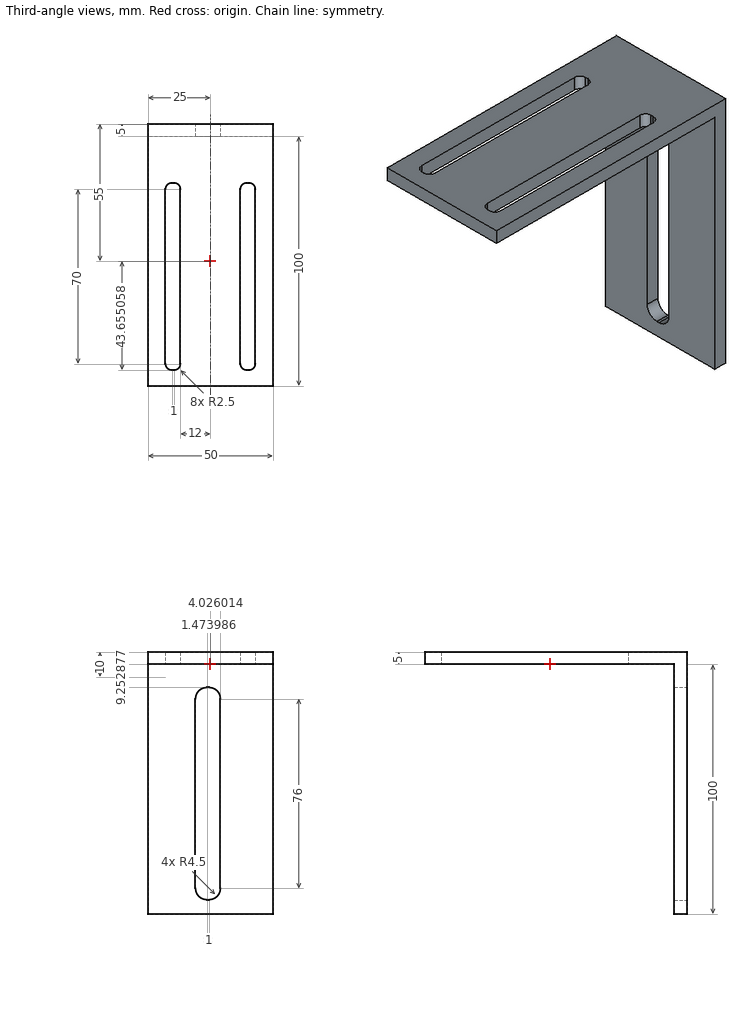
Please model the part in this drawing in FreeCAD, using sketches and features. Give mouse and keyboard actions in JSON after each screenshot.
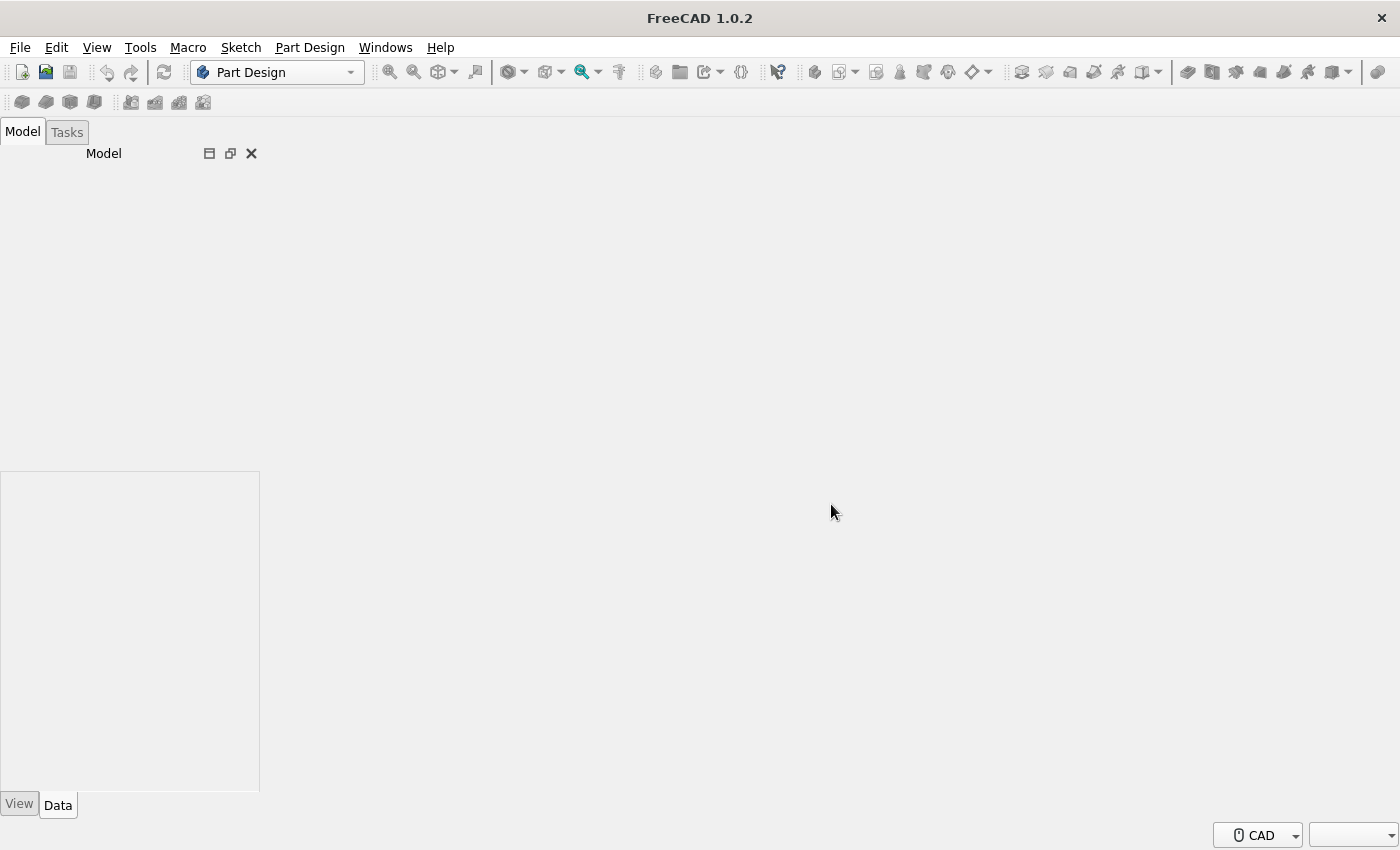
{"action": "left_click", "coordinate": [22, 72]}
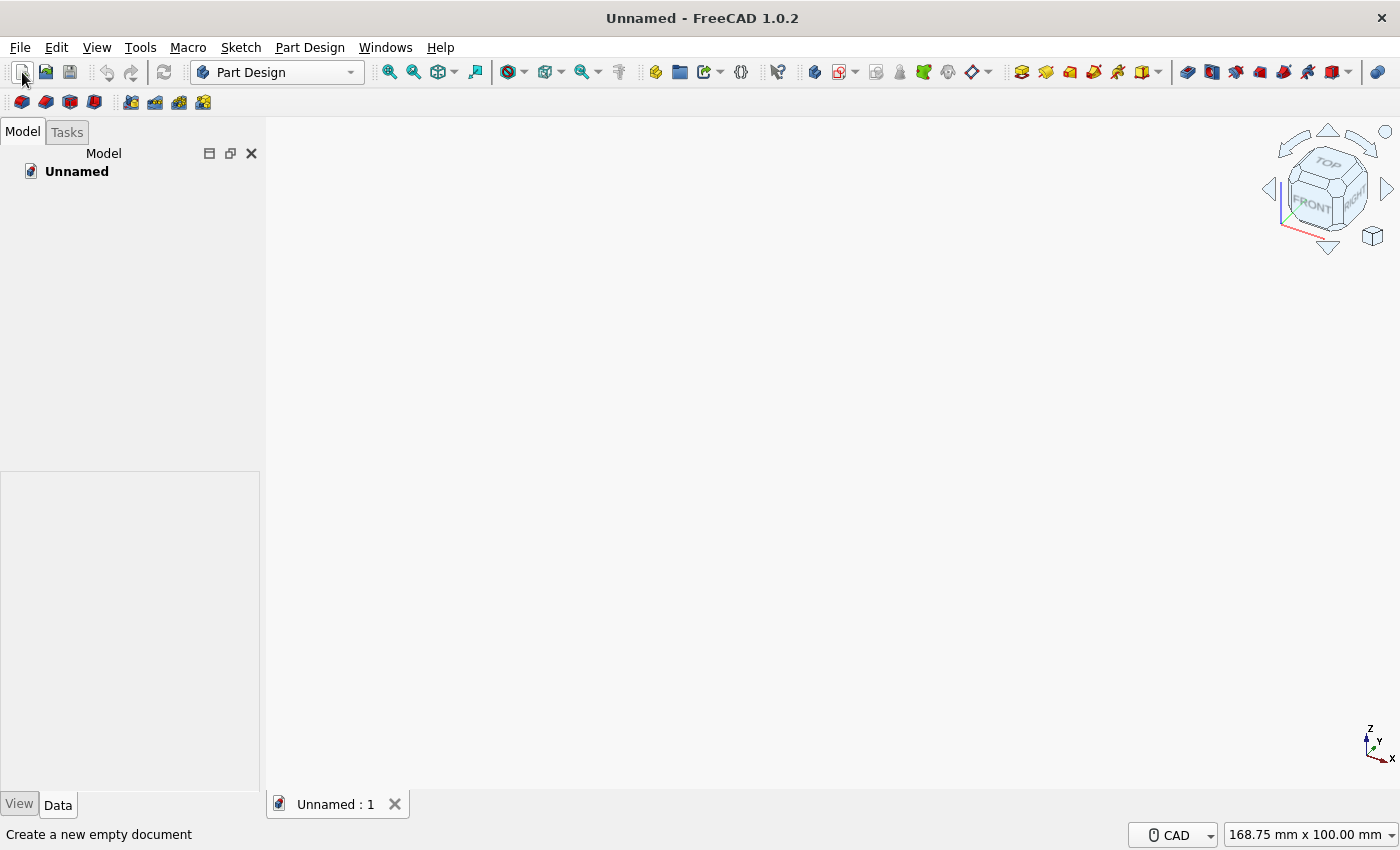
{"action": "left_click", "coordinate": [840, 72]}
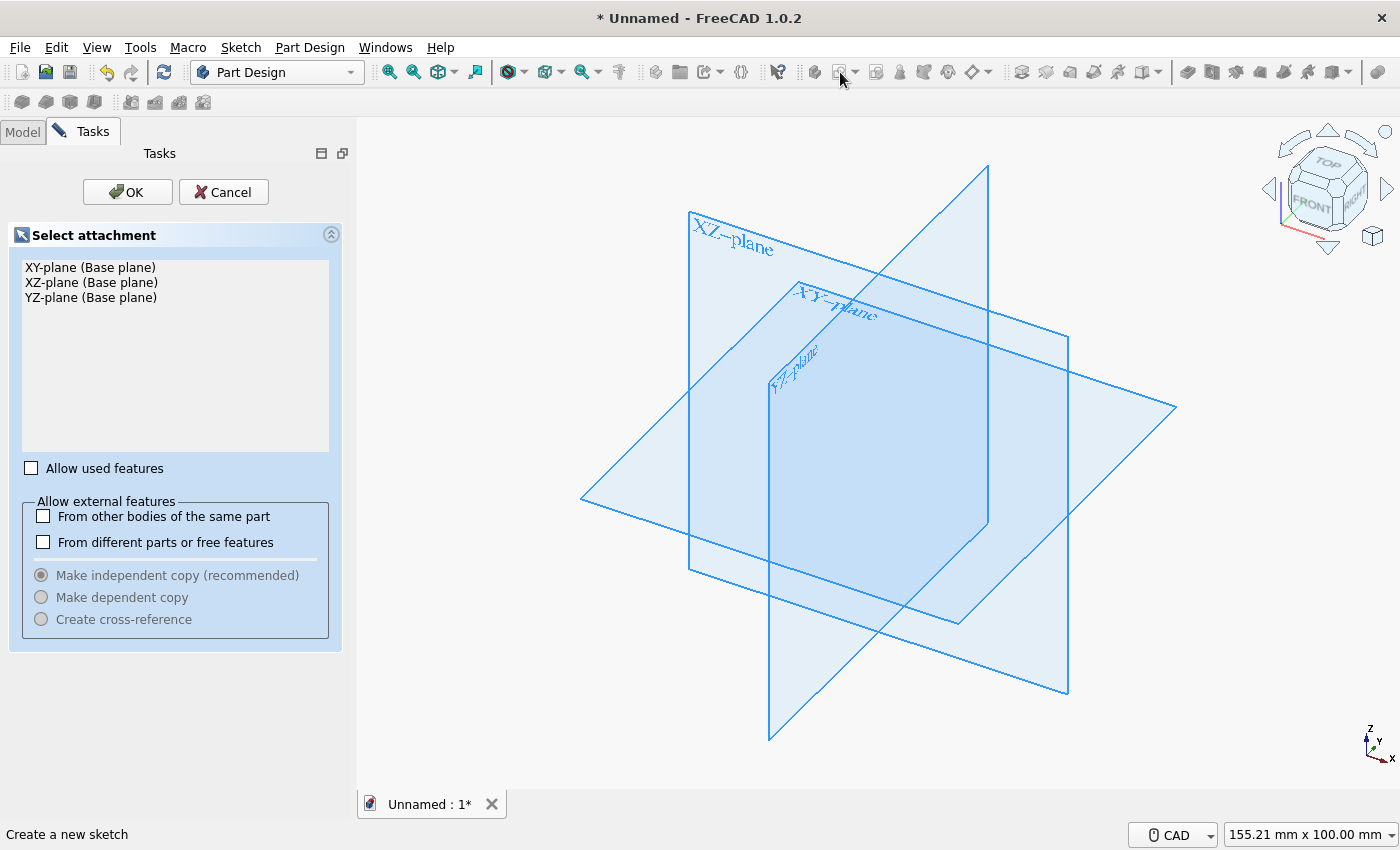
{"action": "left_click", "coordinate": [82, 268]}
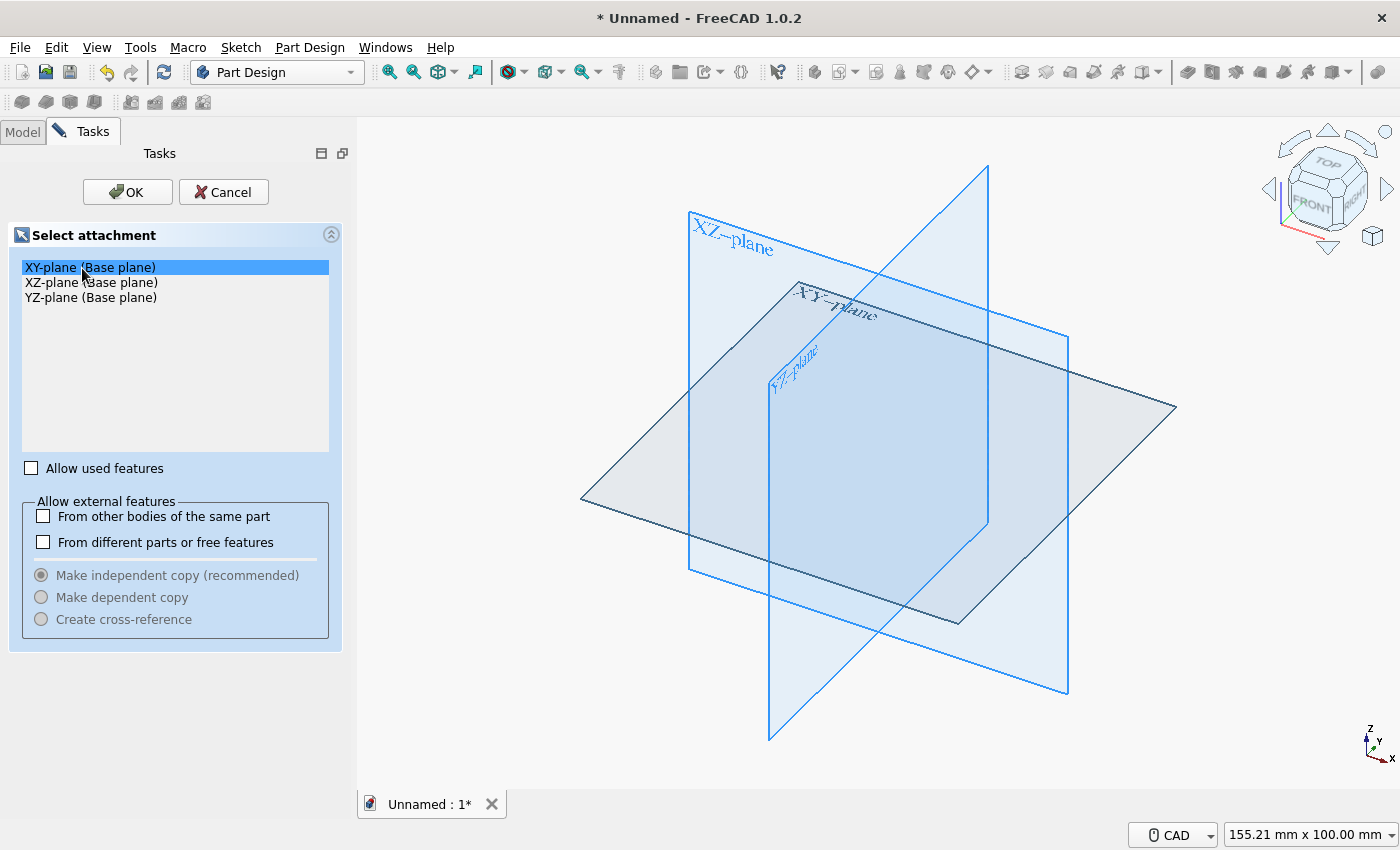
{"action": "left_click", "coordinate": [128, 192]}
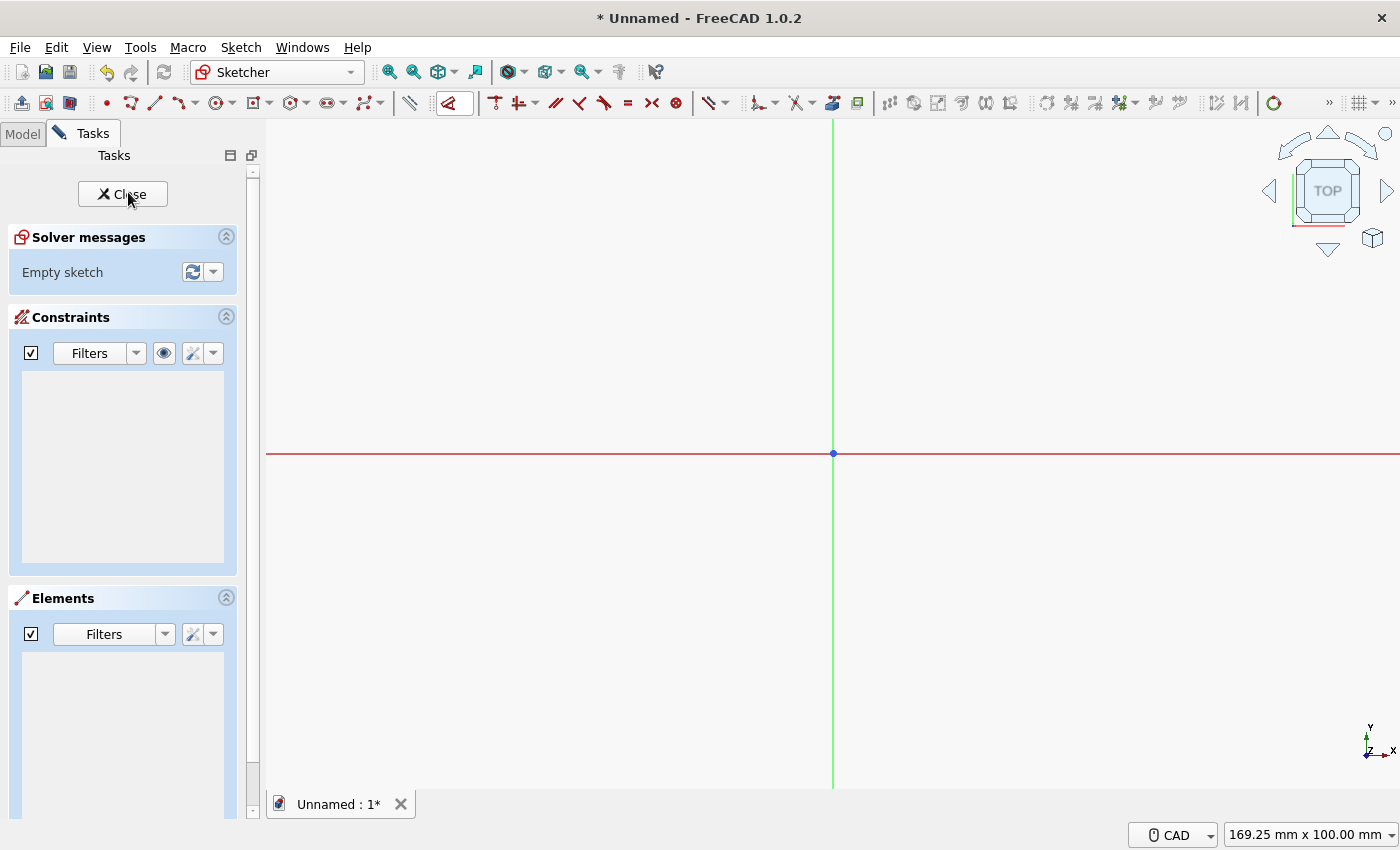
{"action": "scroll", "coordinate": [625, 454], "scroll_direction": "down", "scroll_amount": 2}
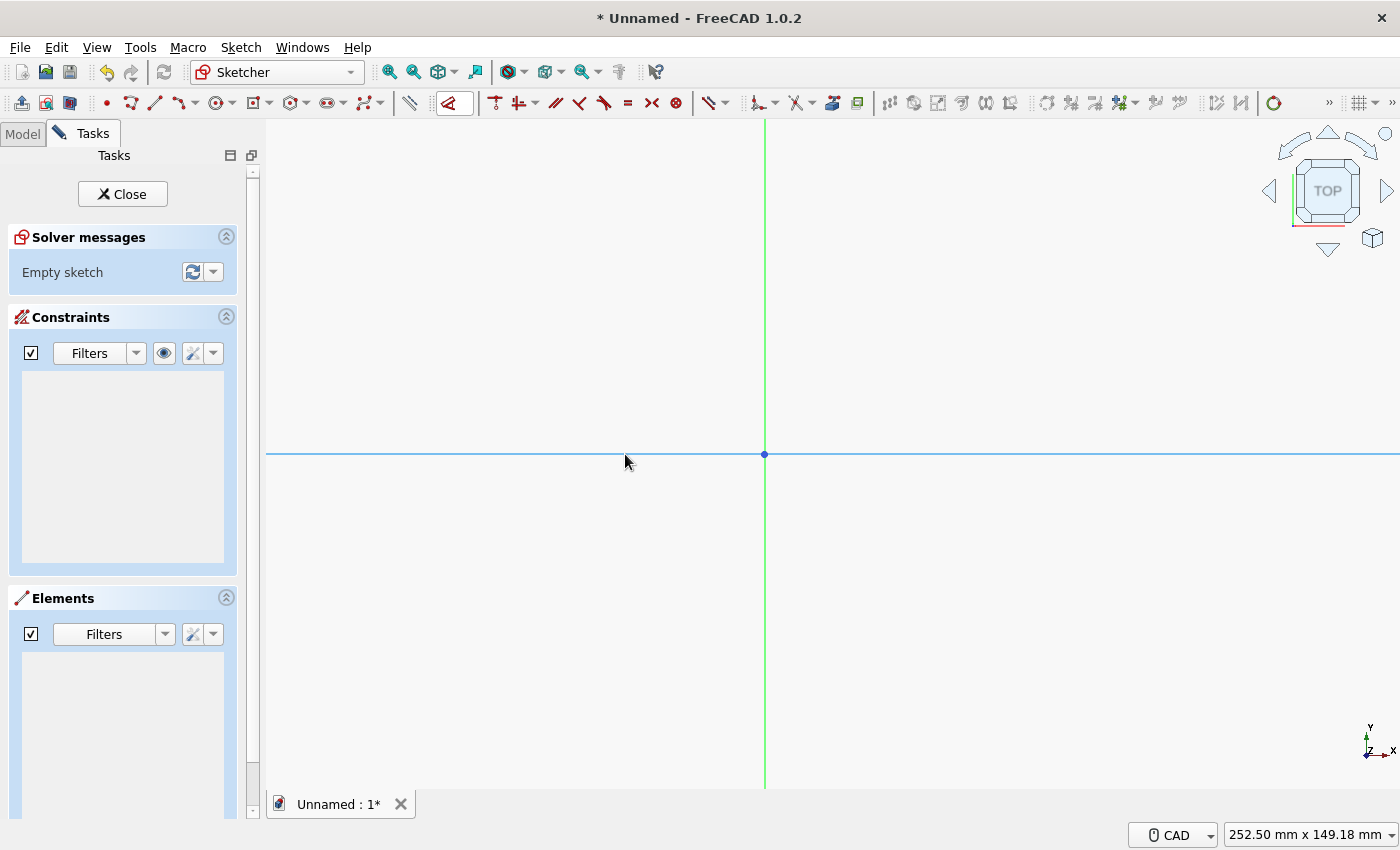
{"action": "key", "text": "g v"}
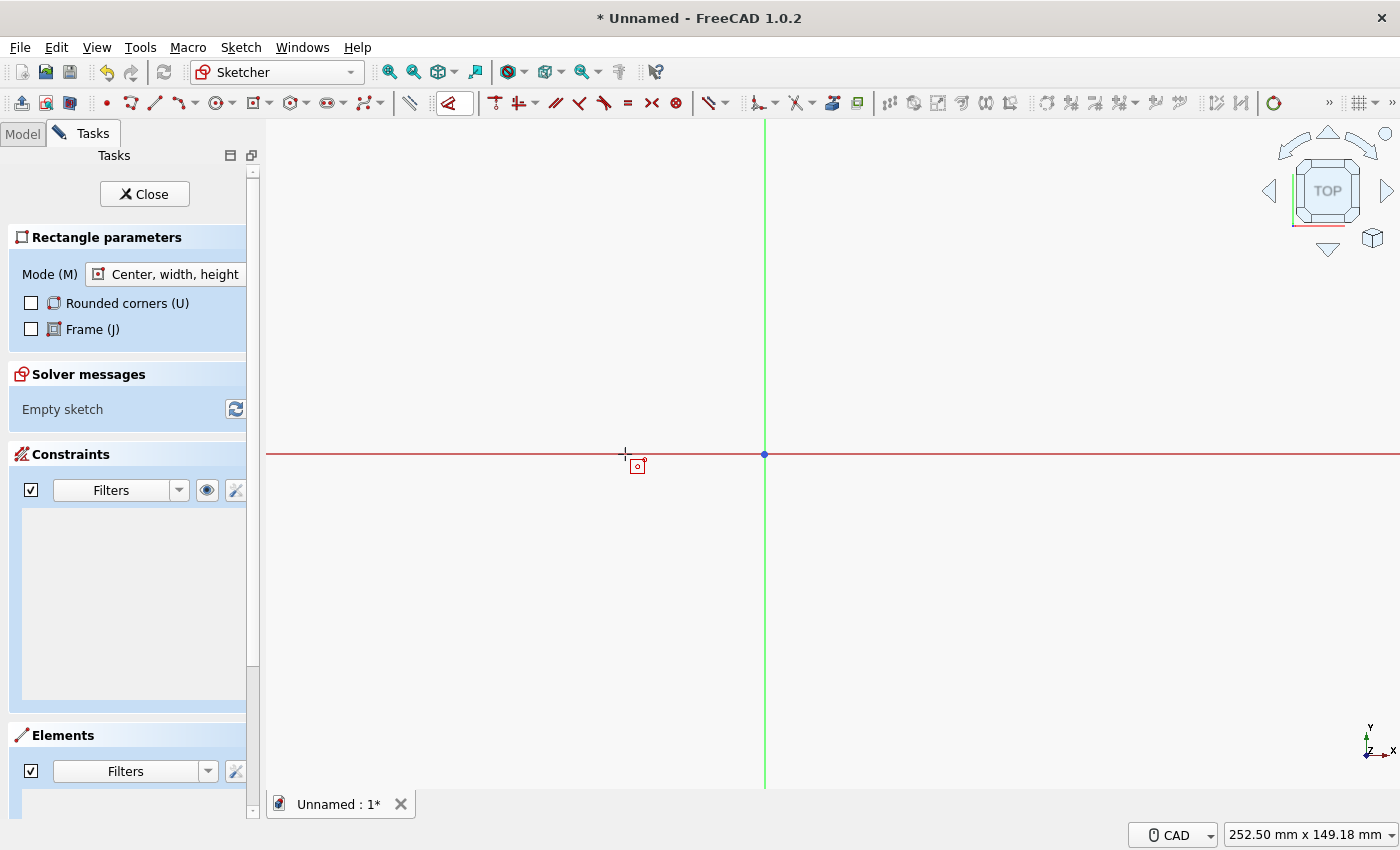
{"action": "left_click", "coordinate": [765, 454]}
{"action": "left_click", "coordinate": [877, 230]}
{"action": "key", "text": "Escape"}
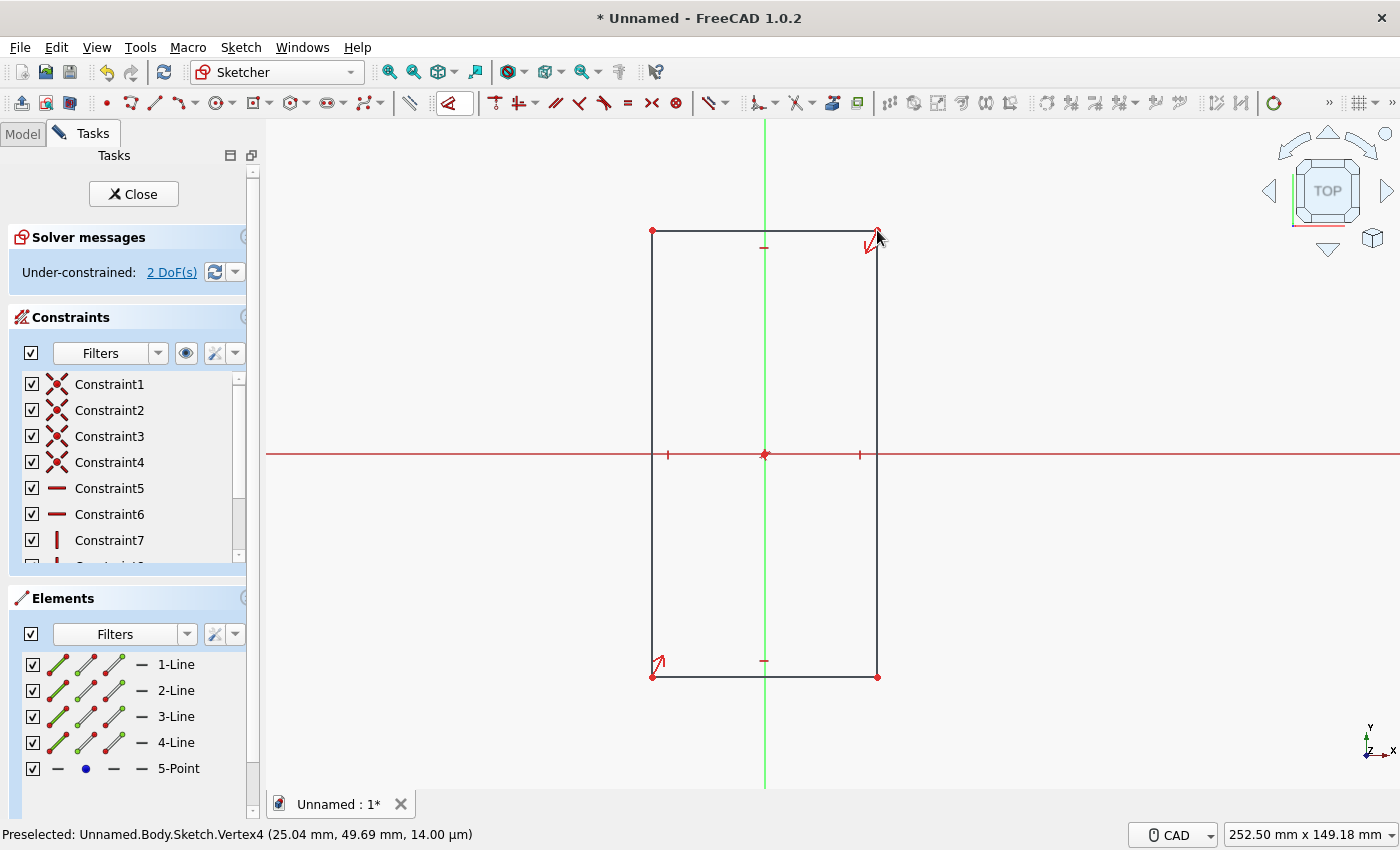
{"action": "left_click", "coordinate": [720, 677]}